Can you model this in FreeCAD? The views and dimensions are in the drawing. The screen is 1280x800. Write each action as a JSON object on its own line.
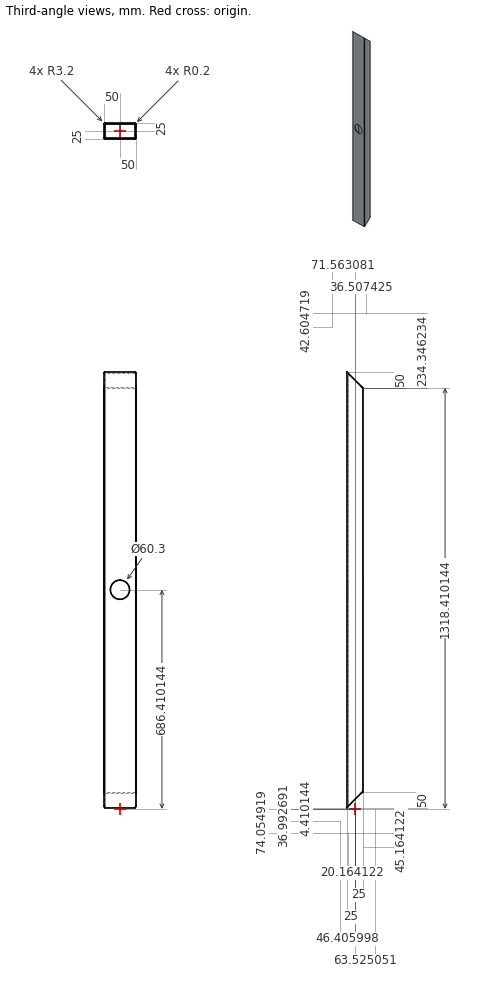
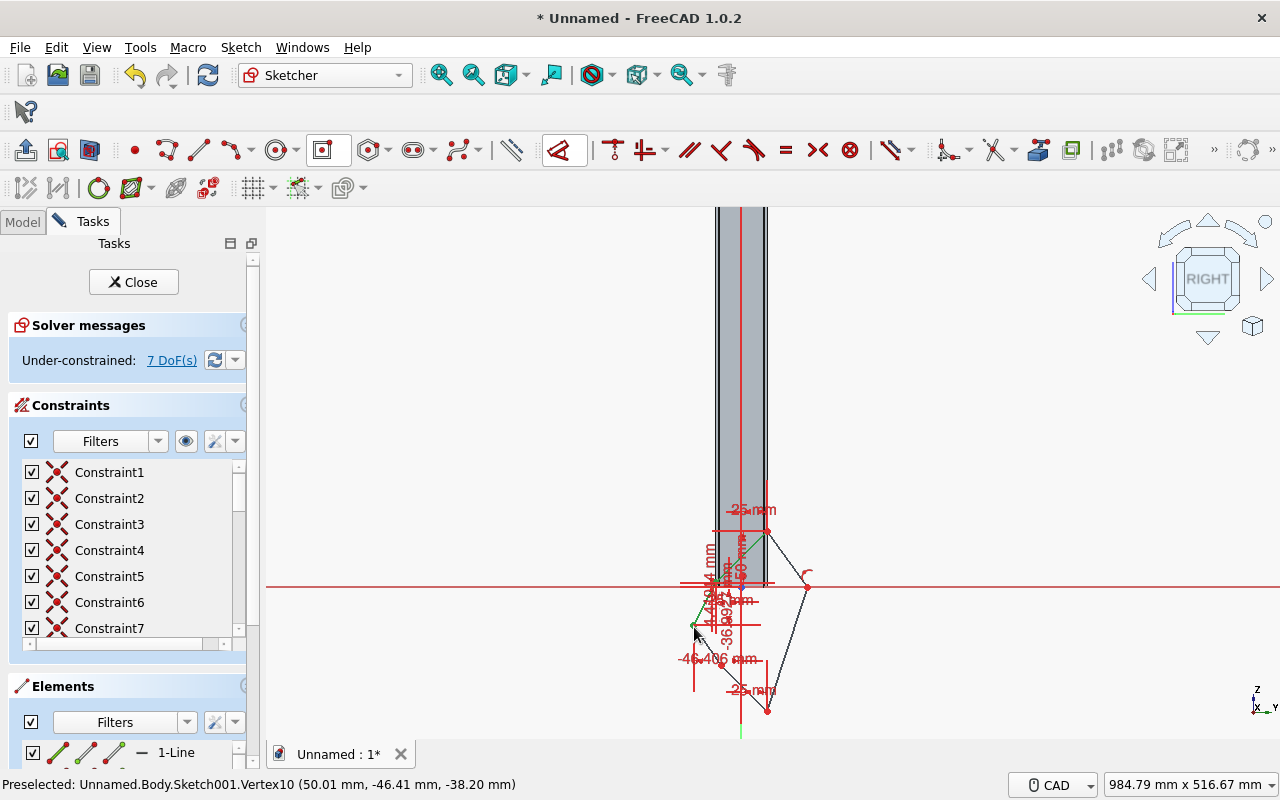
{"action": "scroll", "coordinate": [721, 665], "scroll_direction": "up", "scroll_amount": 4}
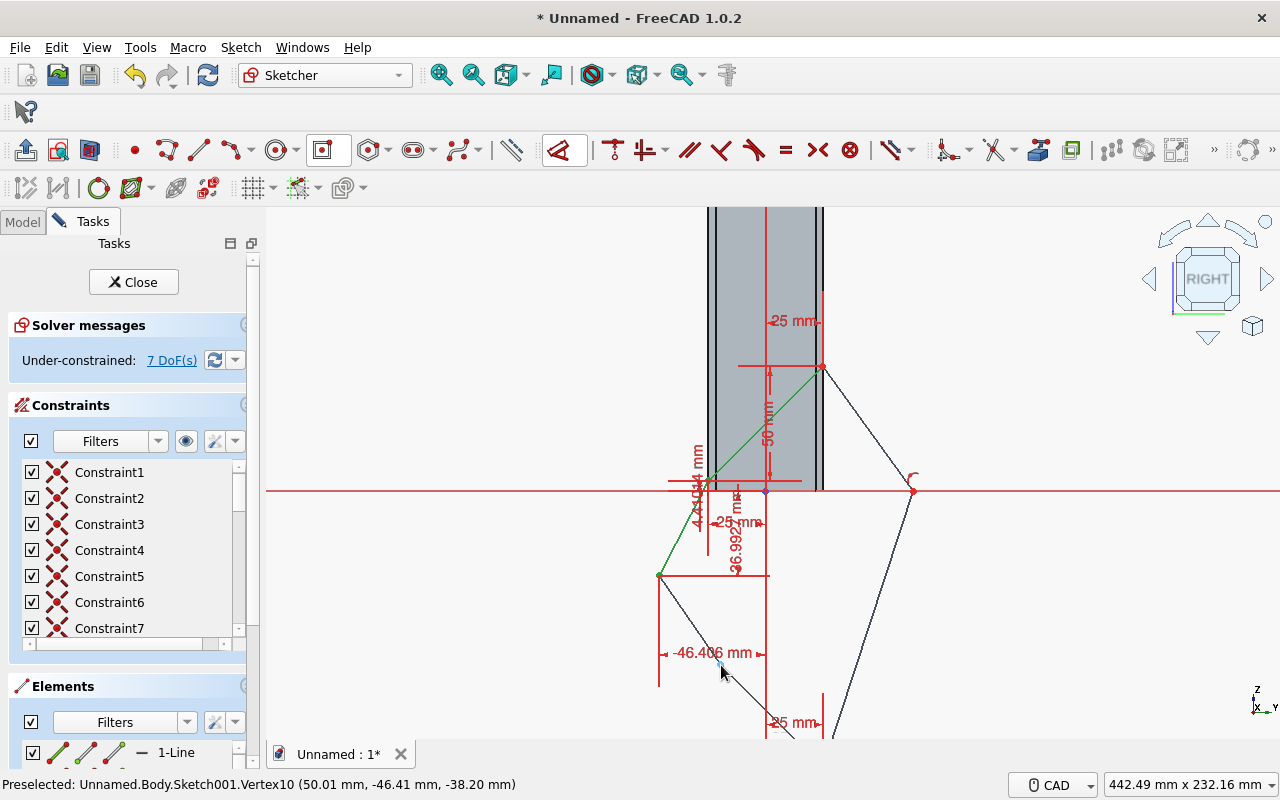
{"action": "left_click", "coordinate": [721, 665]}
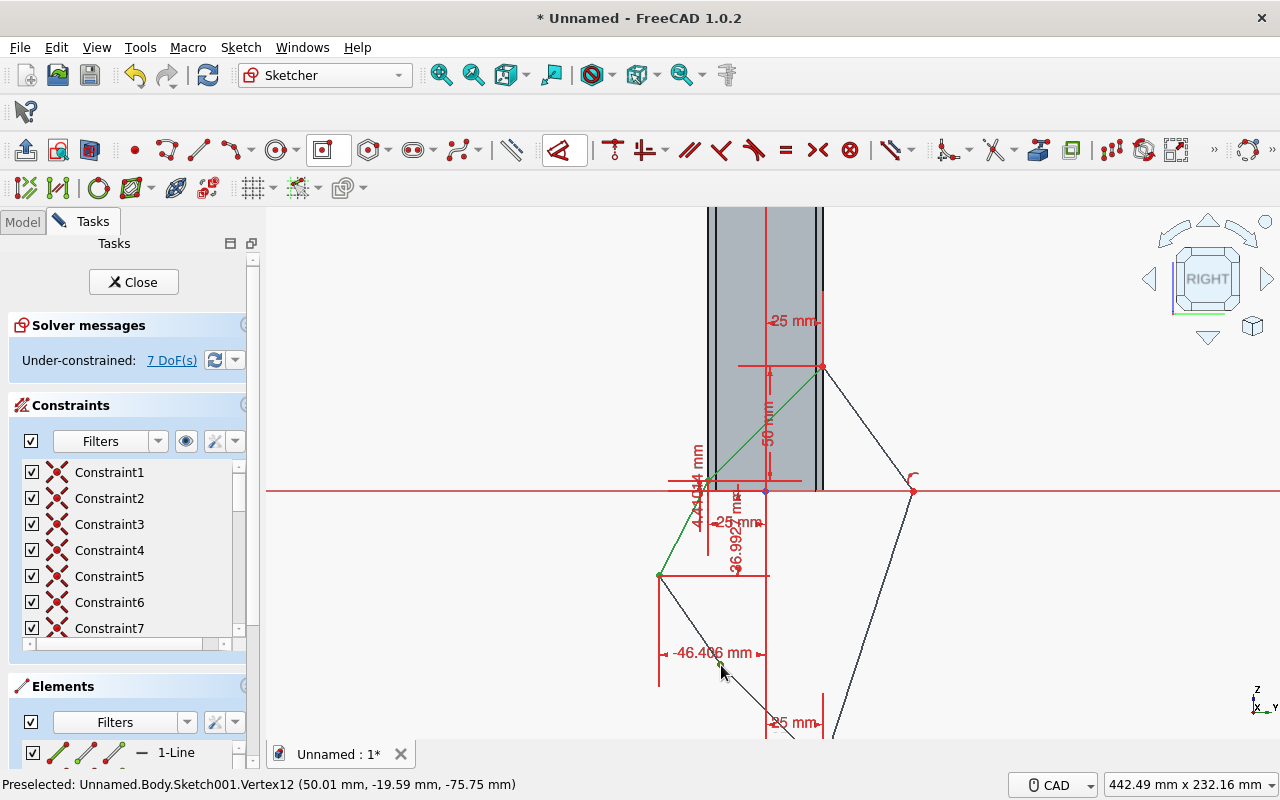
{"action": "left_click", "coordinate": [582, 150]}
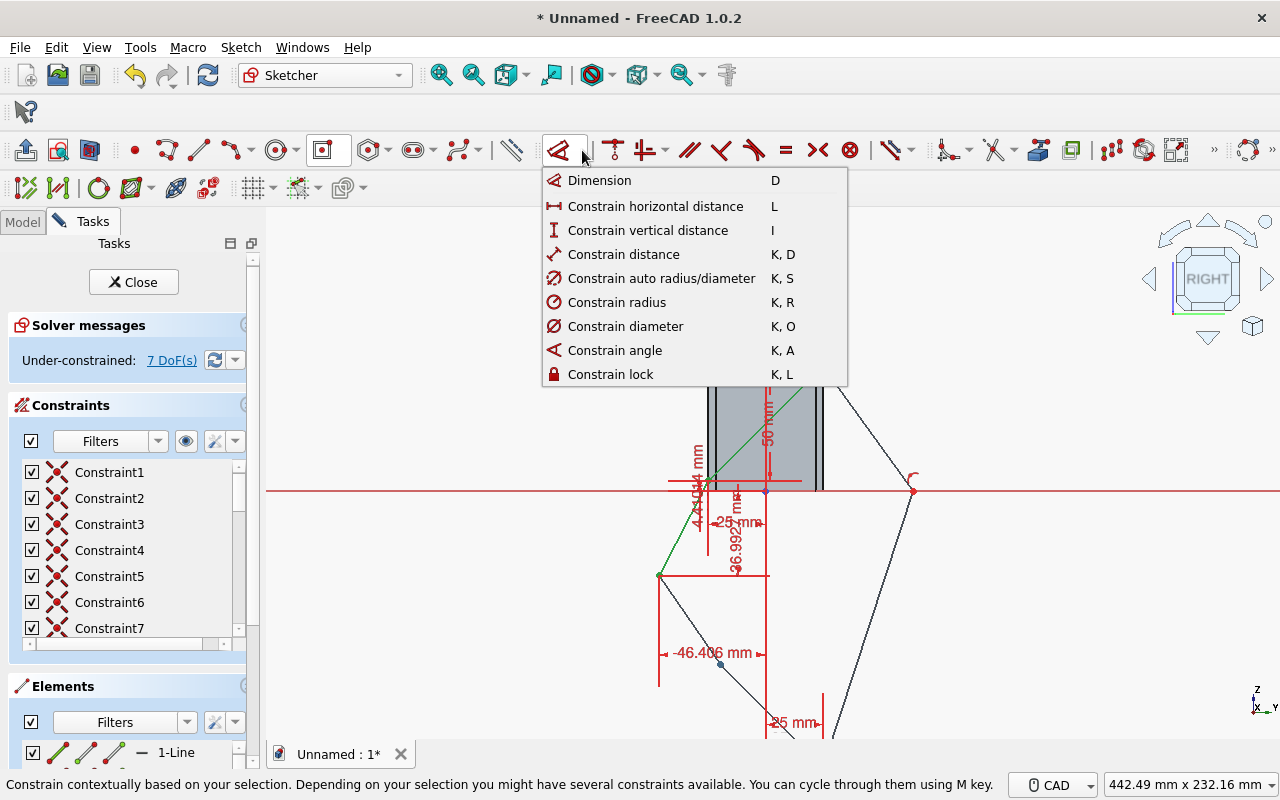
{"action": "left_click", "coordinate": [695, 206]}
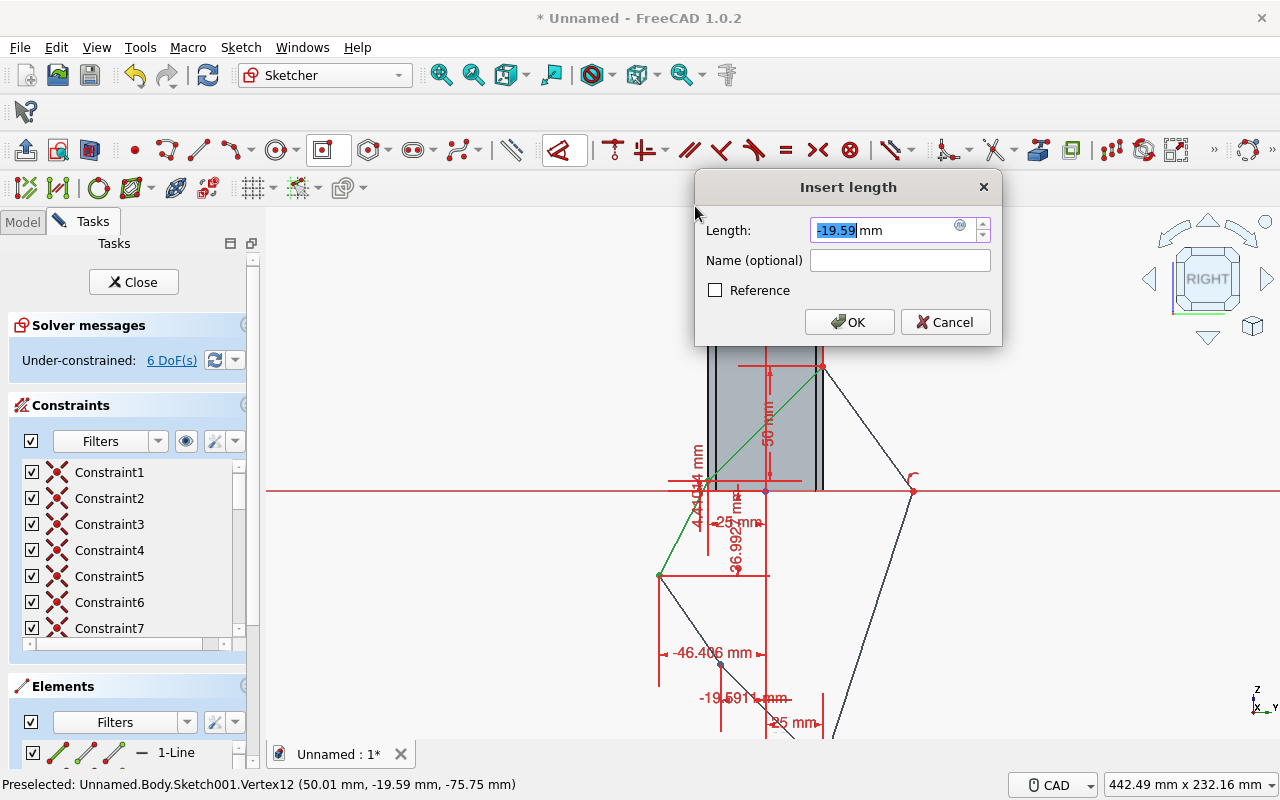
{"action": "type", "text": "-20.164122"}
{"action": "key", "text": "Return"}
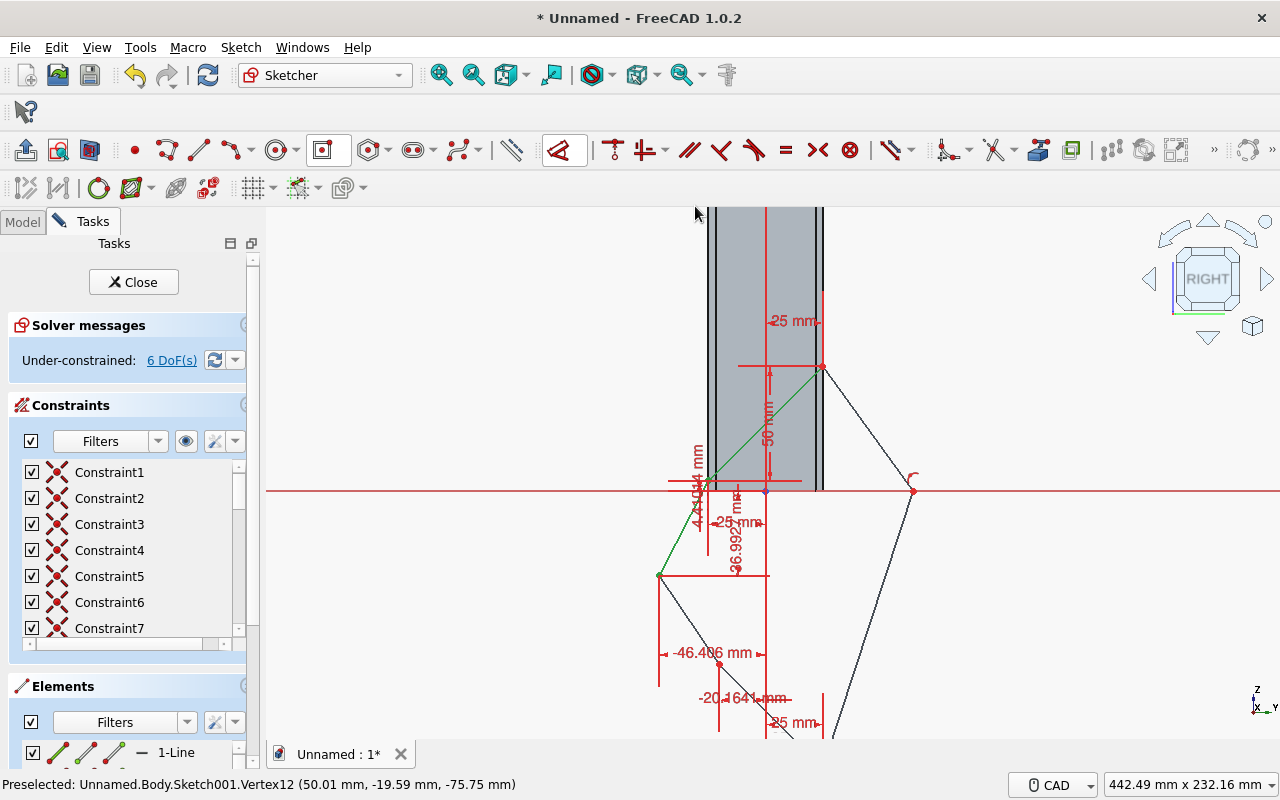
{"action": "scroll", "coordinate": [699, 635], "scroll_direction": "down", "scroll_amount": 12}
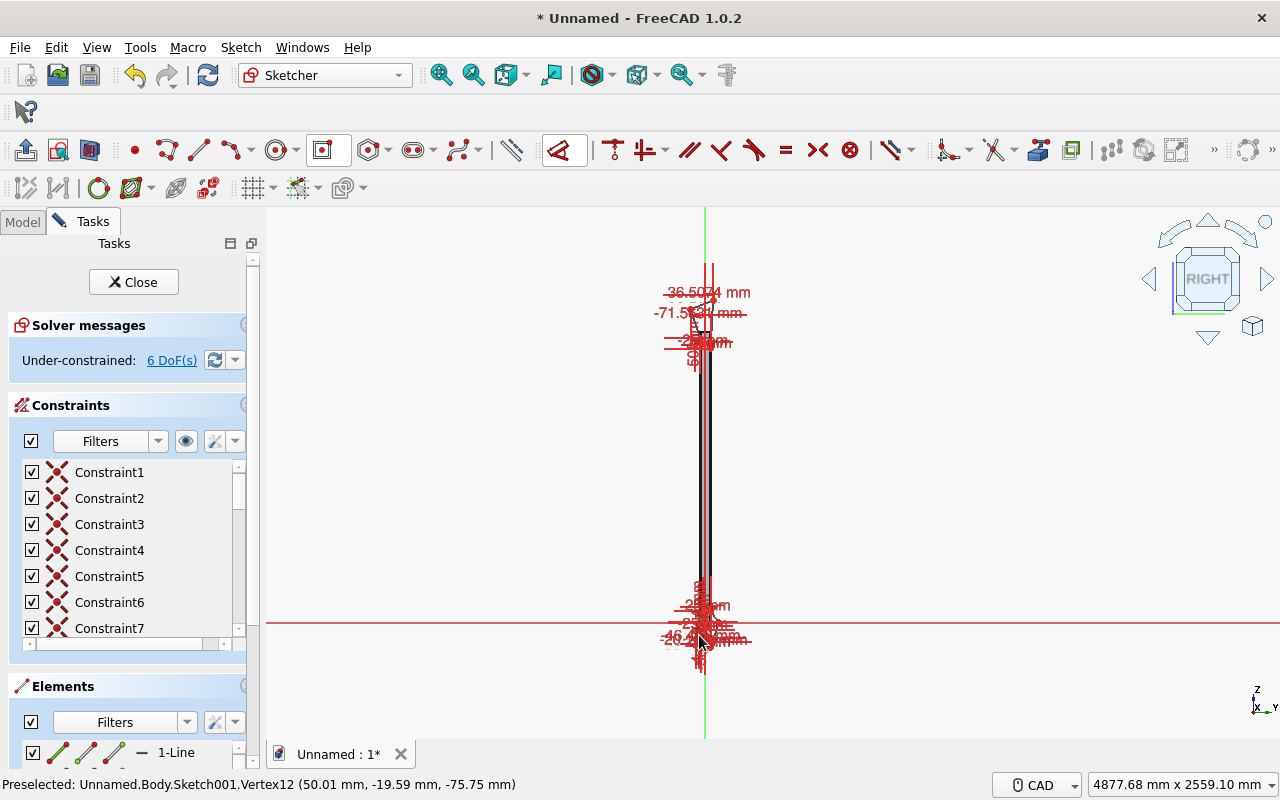
{"action": "scroll", "coordinate": [701, 638], "scroll_direction": "up", "scroll_amount": 5}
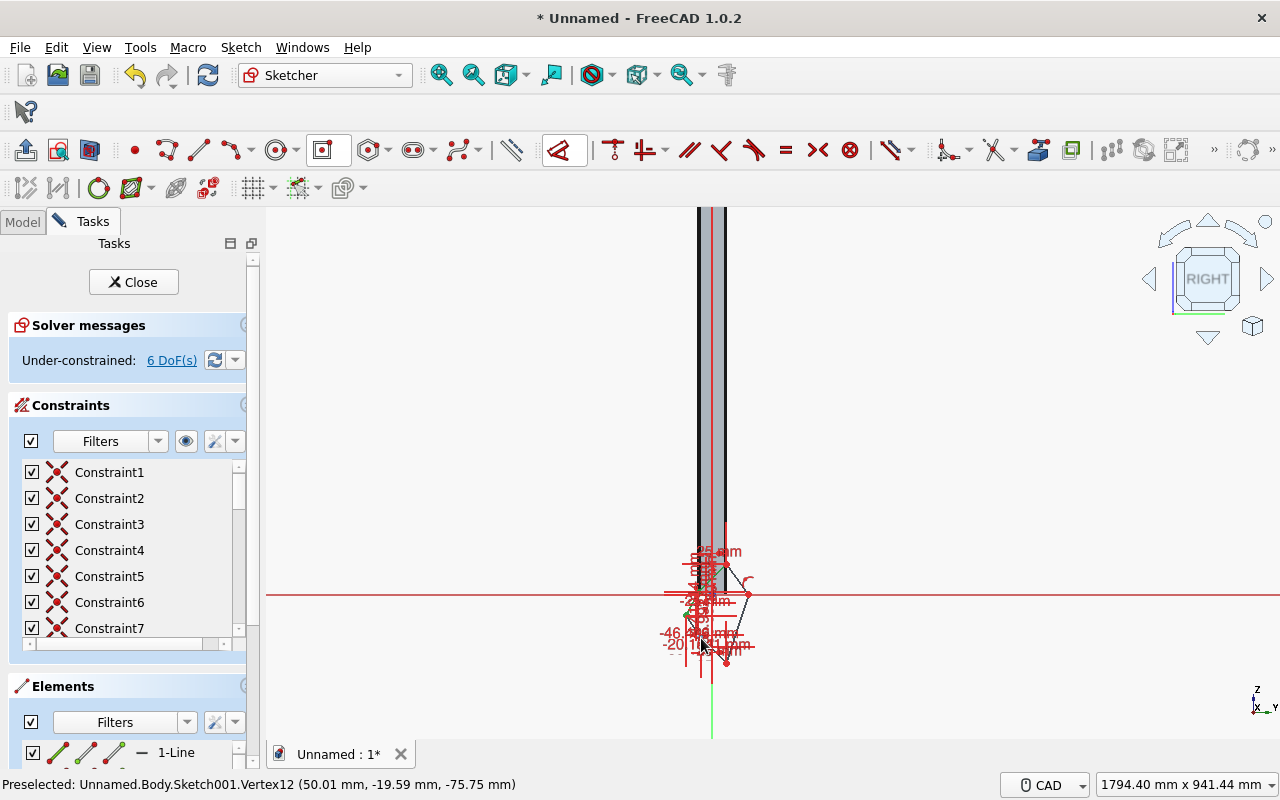
{"action": "left_click", "coordinate": [701, 638]}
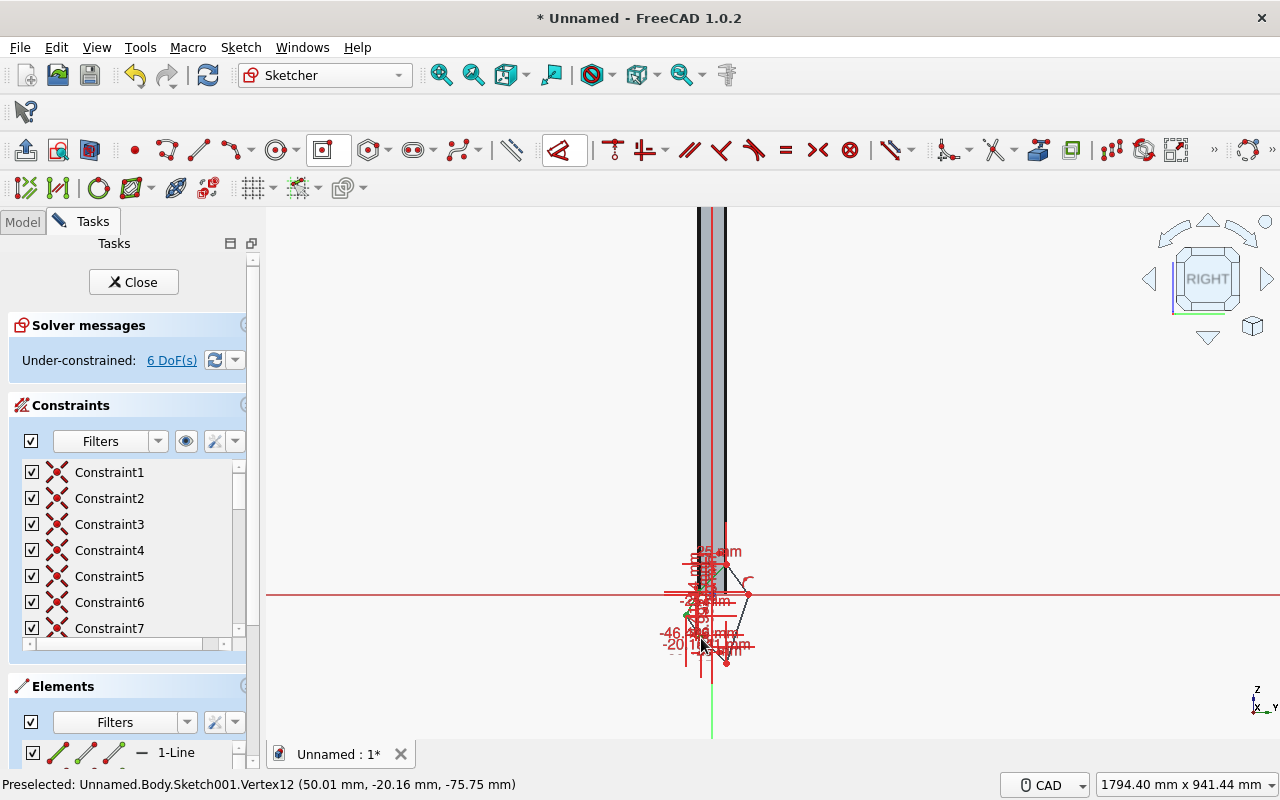
{"action": "left_click", "coordinate": [582, 150]}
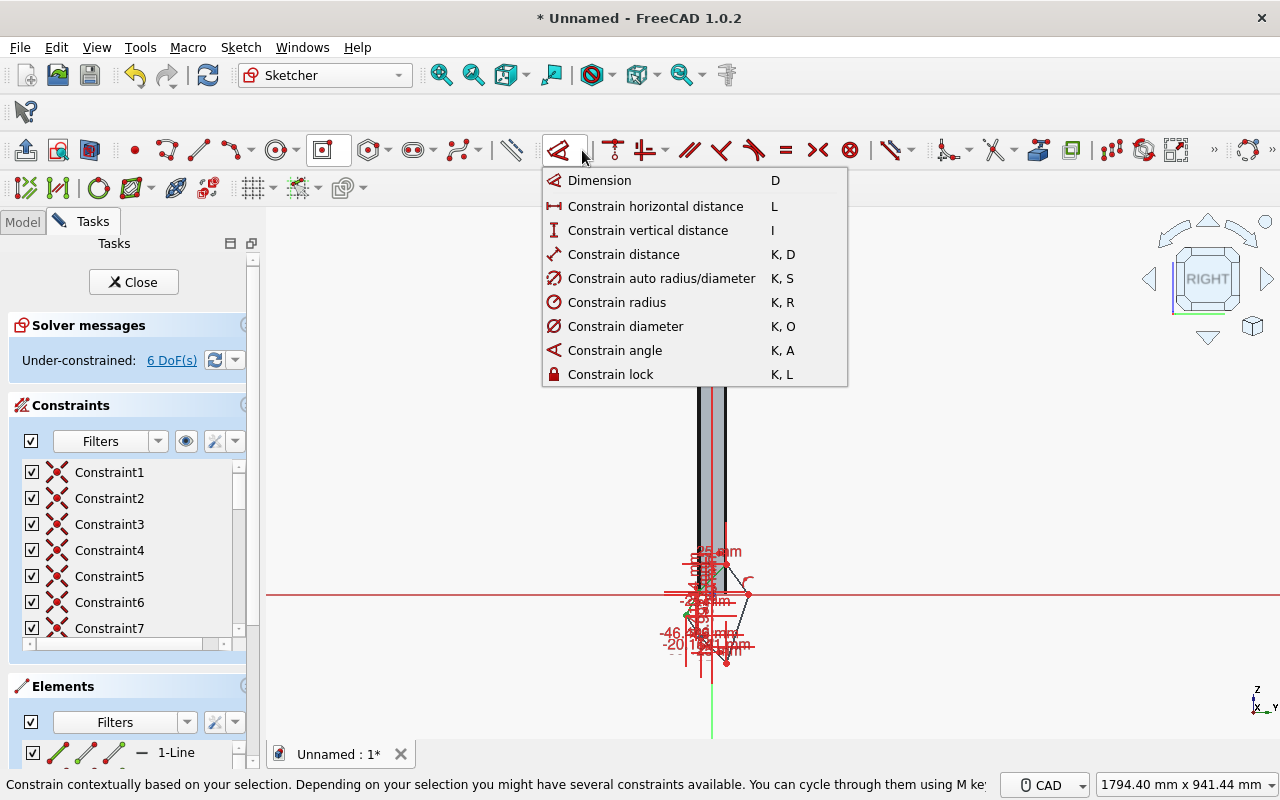
{"action": "left_click", "coordinate": [695, 230]}